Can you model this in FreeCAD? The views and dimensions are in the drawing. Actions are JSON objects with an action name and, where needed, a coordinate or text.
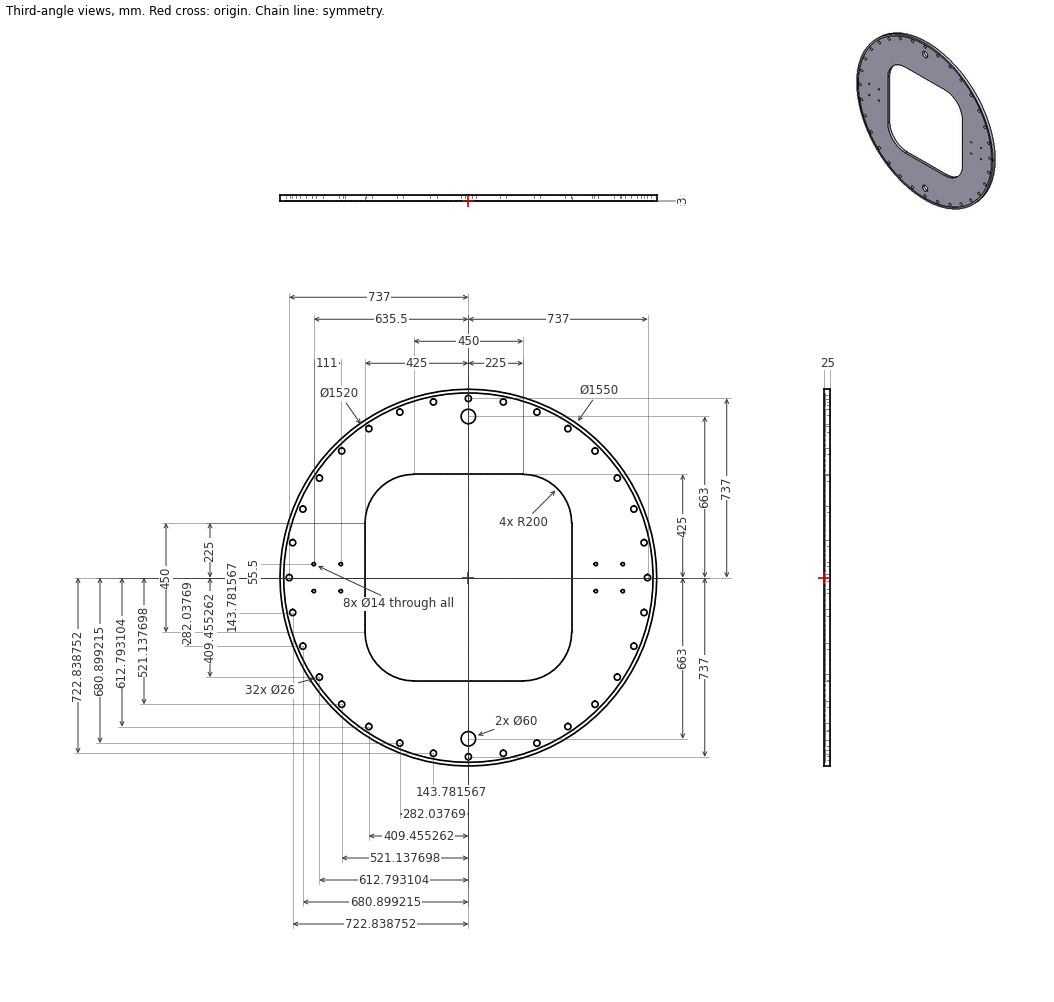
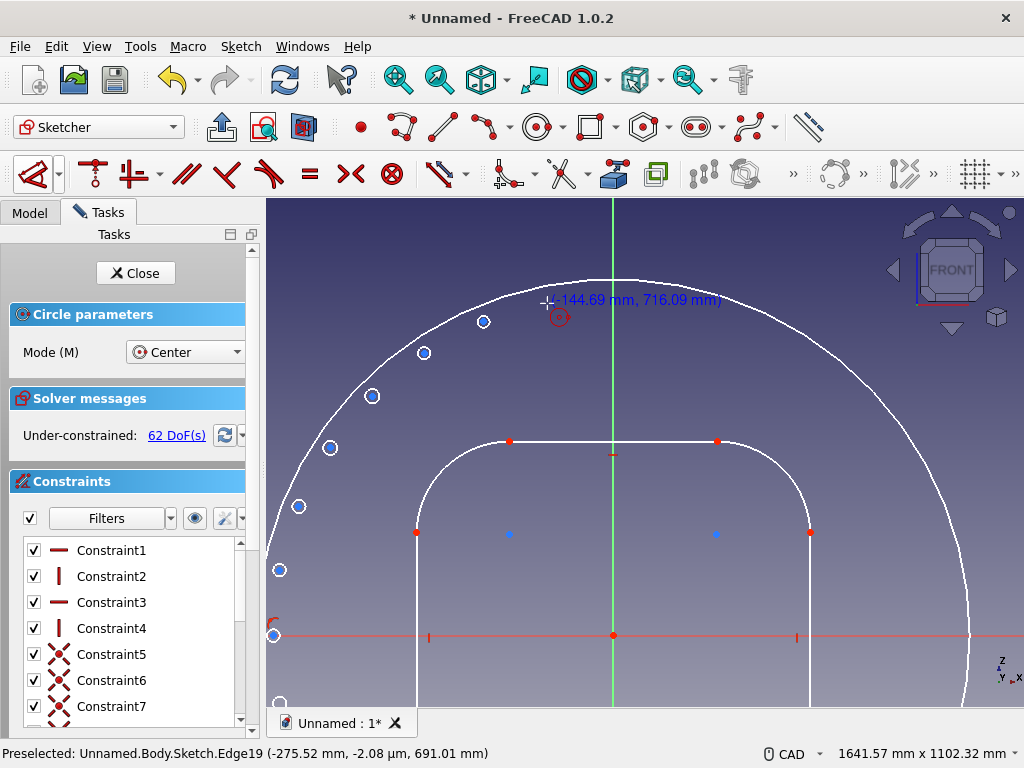
{"action": "left_click", "coordinate": [547, 302]}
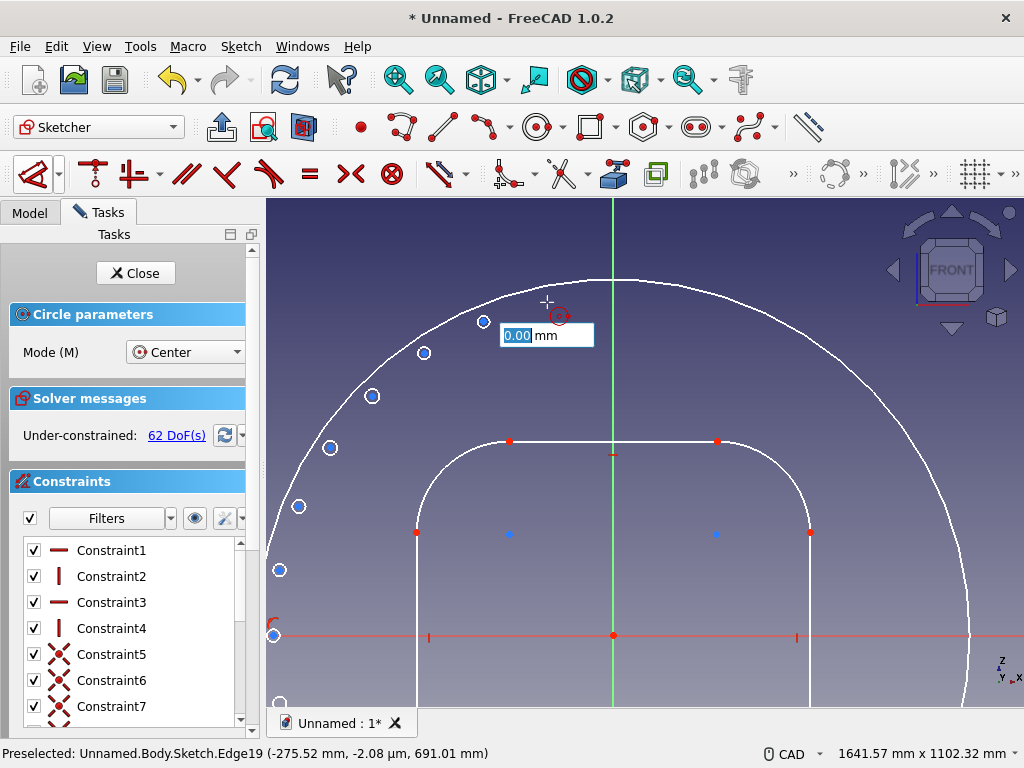
{"action": "scroll", "coordinate": [551, 298], "scroll_direction": "up", "scroll_amount": 5}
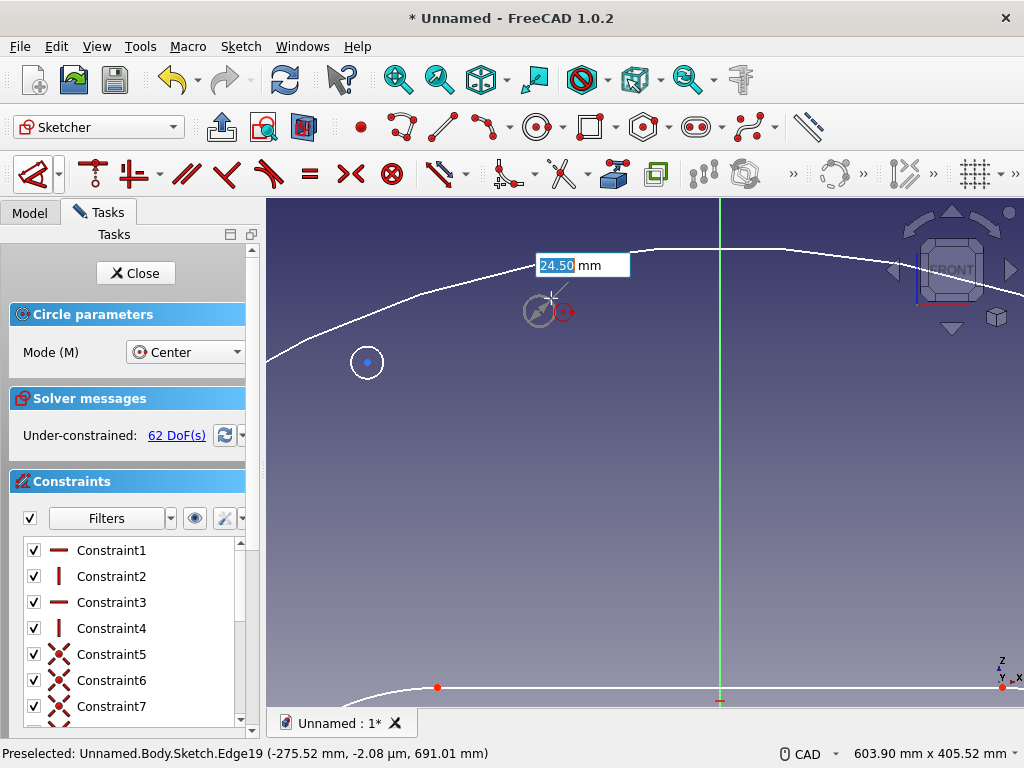
{"action": "left_click", "coordinate": [551, 297]}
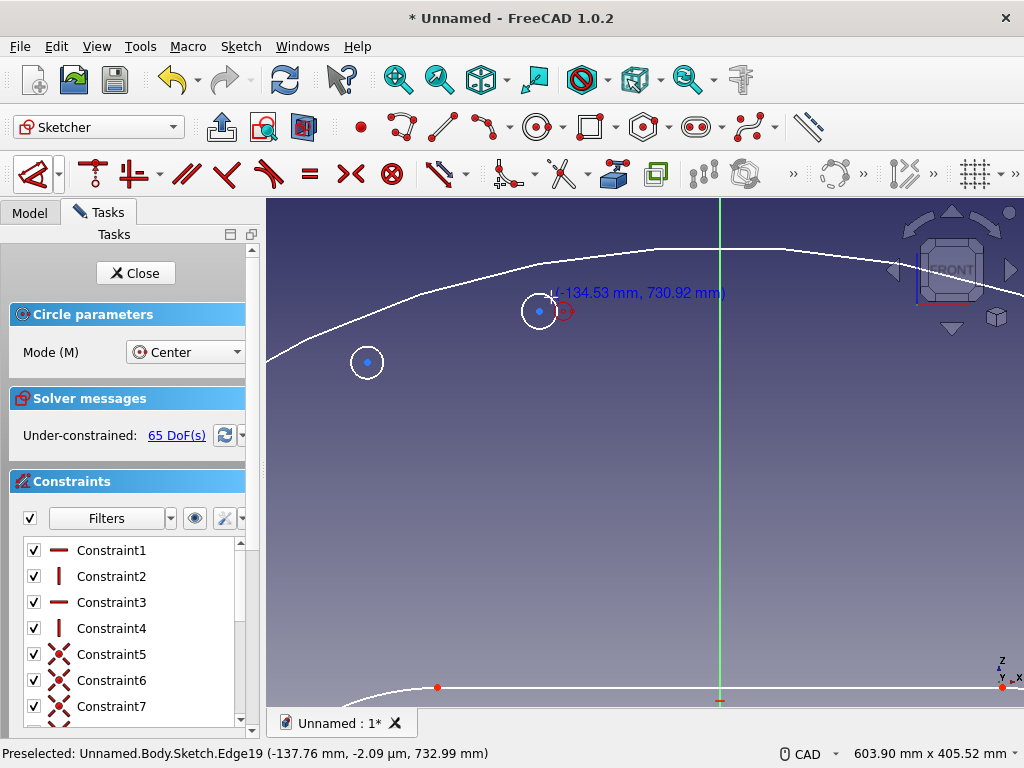
{"action": "scroll", "coordinate": [548, 301], "scroll_direction": "down", "scroll_amount": 9}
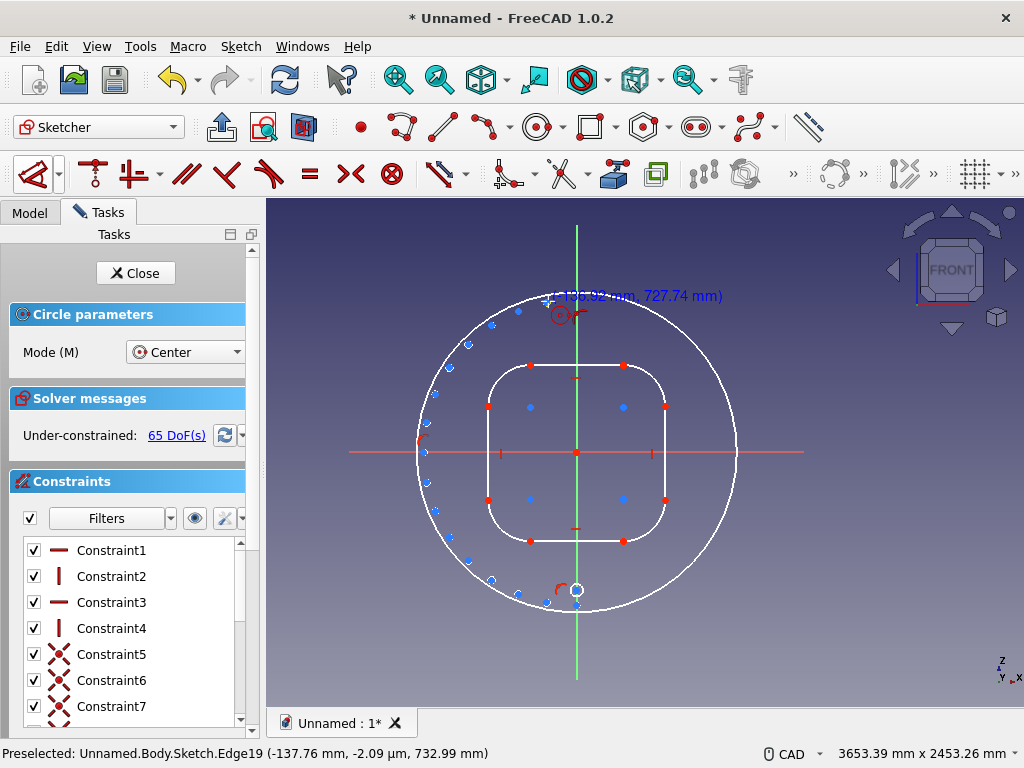
{"action": "scroll", "coordinate": [607, 602], "scroll_direction": "up", "scroll_amount": 11}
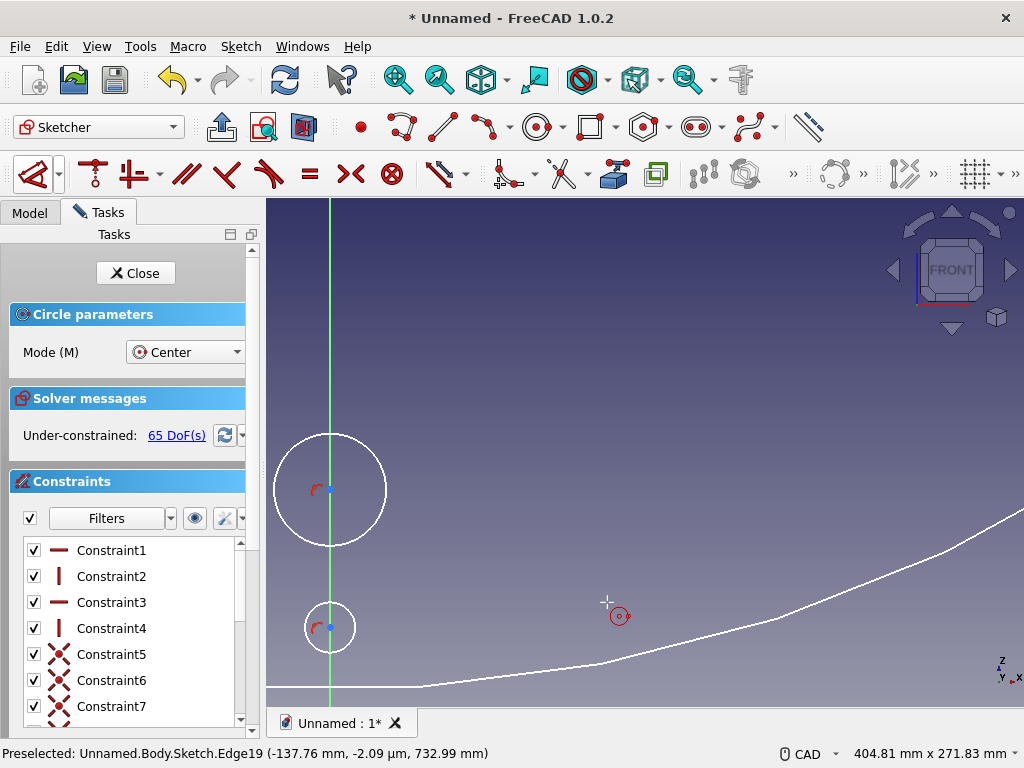
{"action": "scroll", "coordinate": [607, 603], "scroll_direction": "down", "scroll_amount": 11}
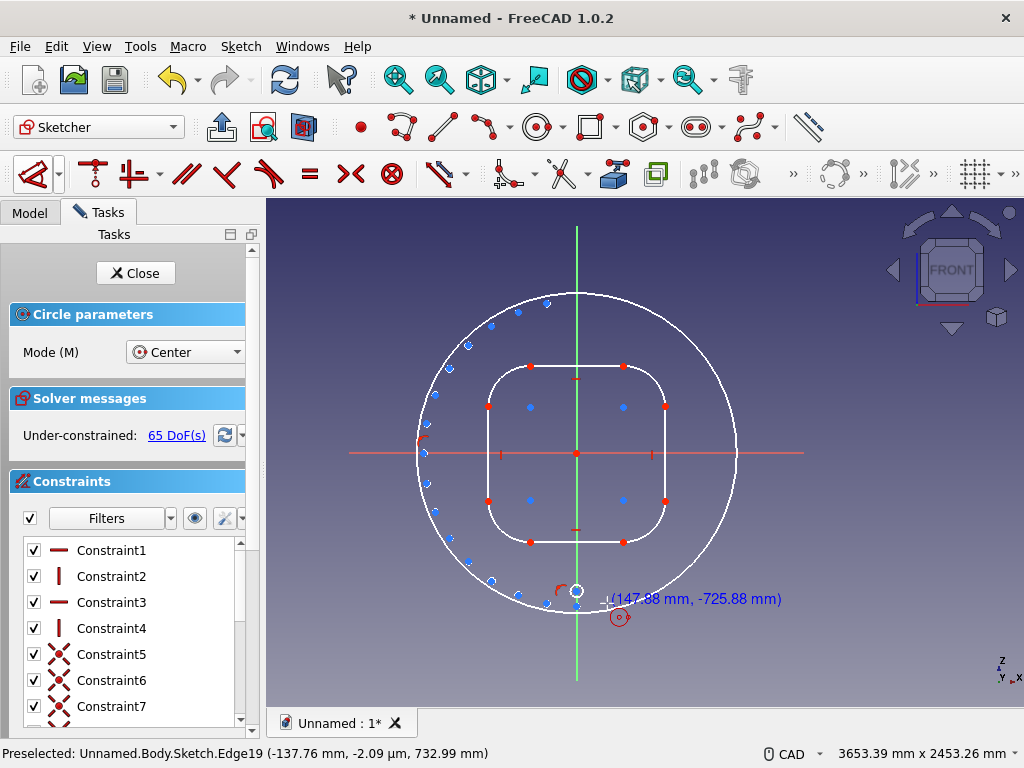
{"action": "scroll", "coordinate": [607, 603], "scroll_direction": "up", "scroll_amount": 4}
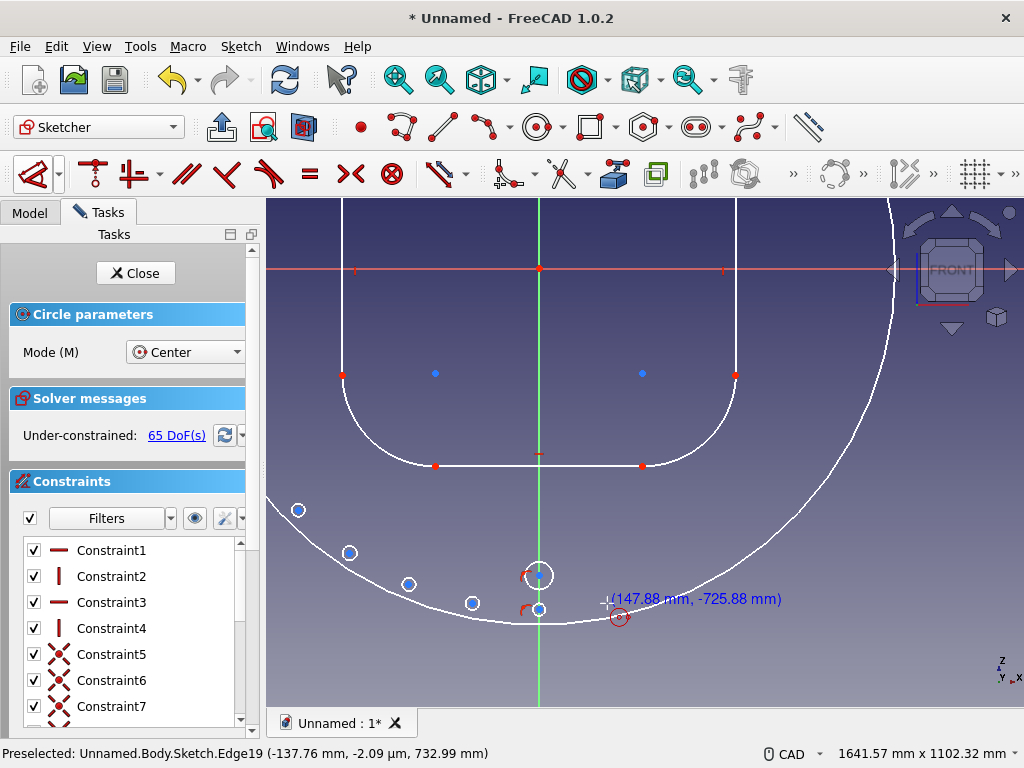
{"action": "left_click", "coordinate": [605, 602]}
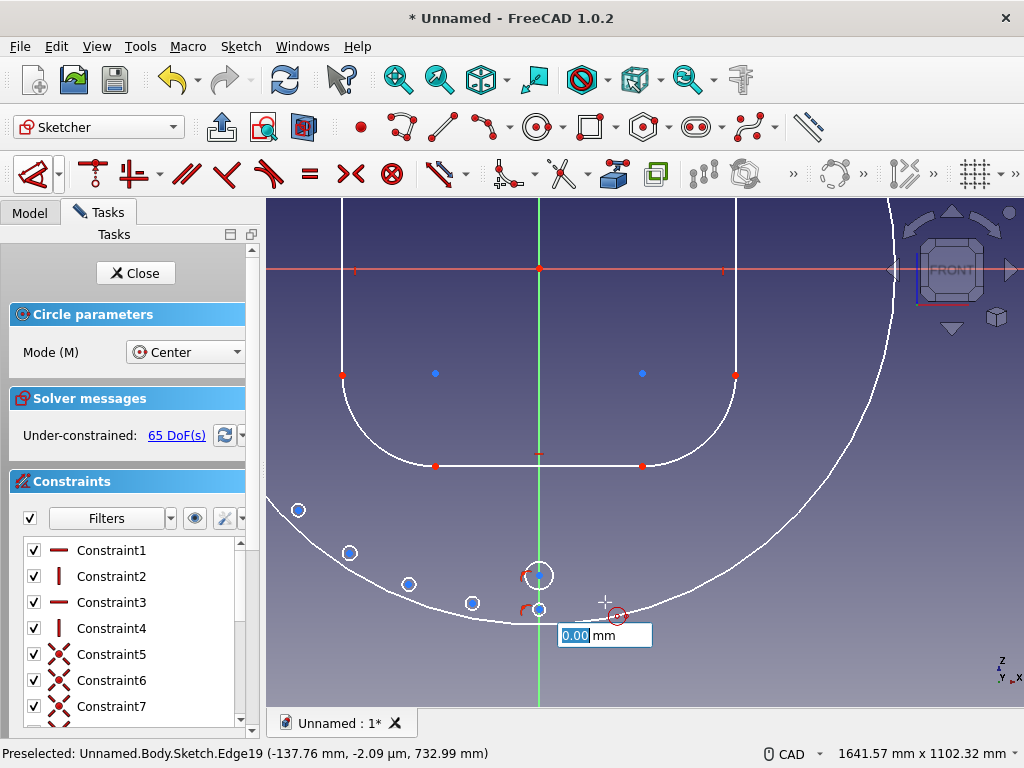
{"action": "scroll", "coordinate": [610, 598], "scroll_direction": "up", "scroll_amount": 5}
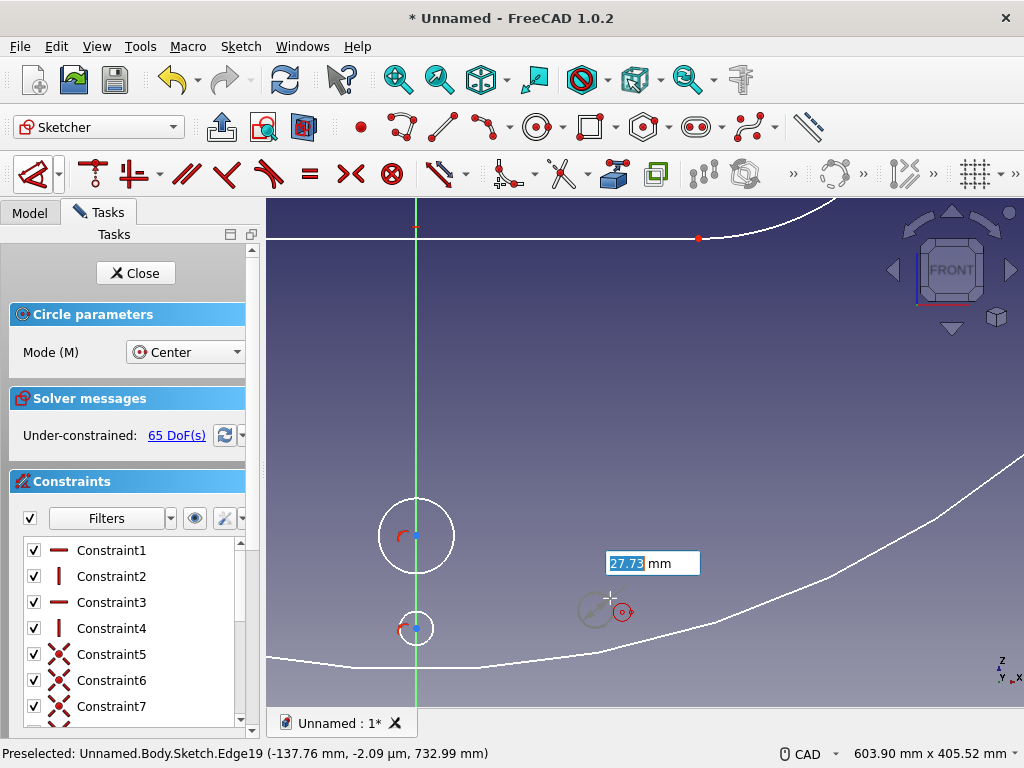
{"action": "left_click", "coordinate": [608, 597]}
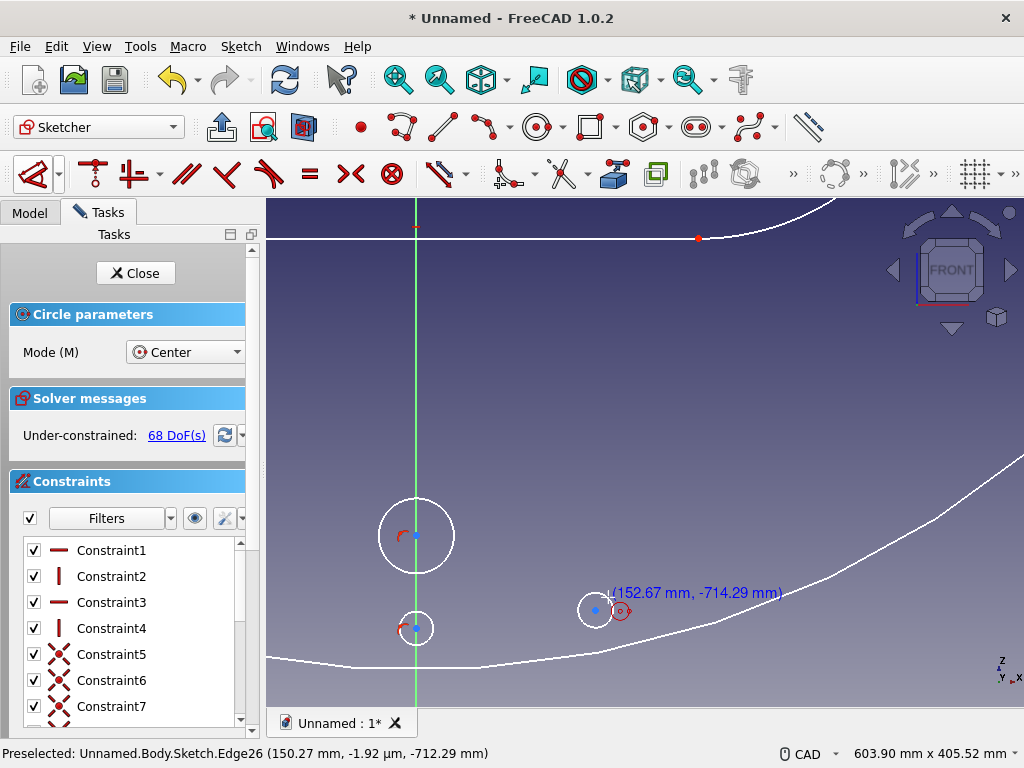
{"action": "scroll", "coordinate": [770, 556], "scroll_direction": "up", "scroll_amount": 2}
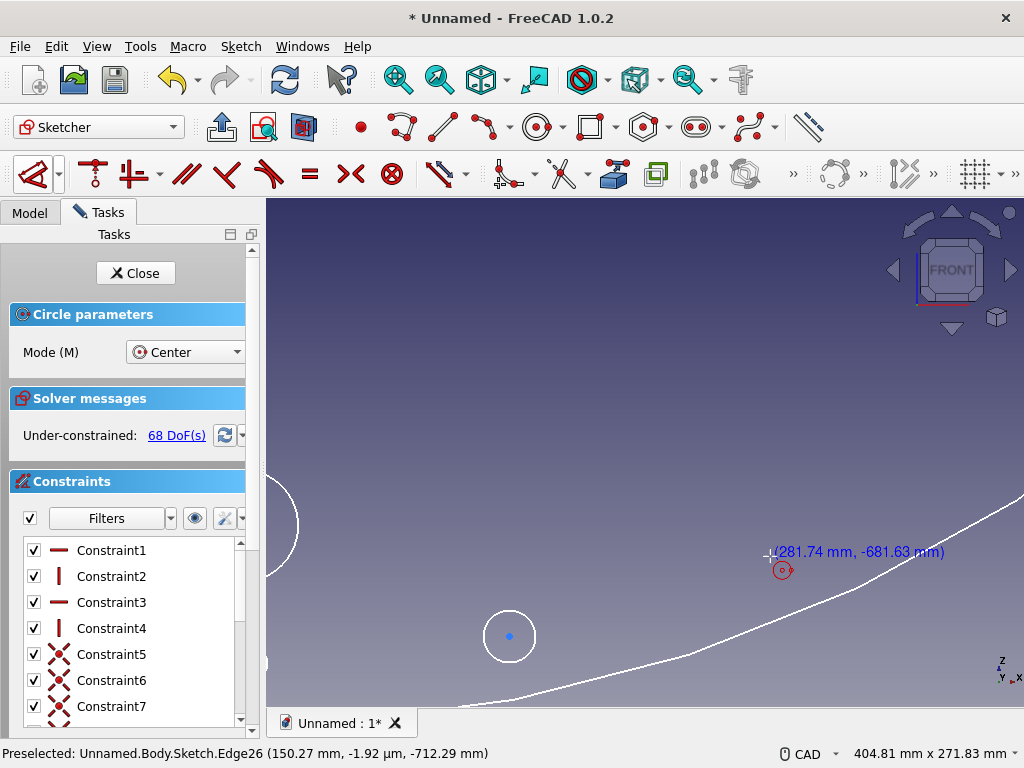
{"action": "scroll", "coordinate": [618, 599], "scroll_direction": "down", "scroll_amount": 11}